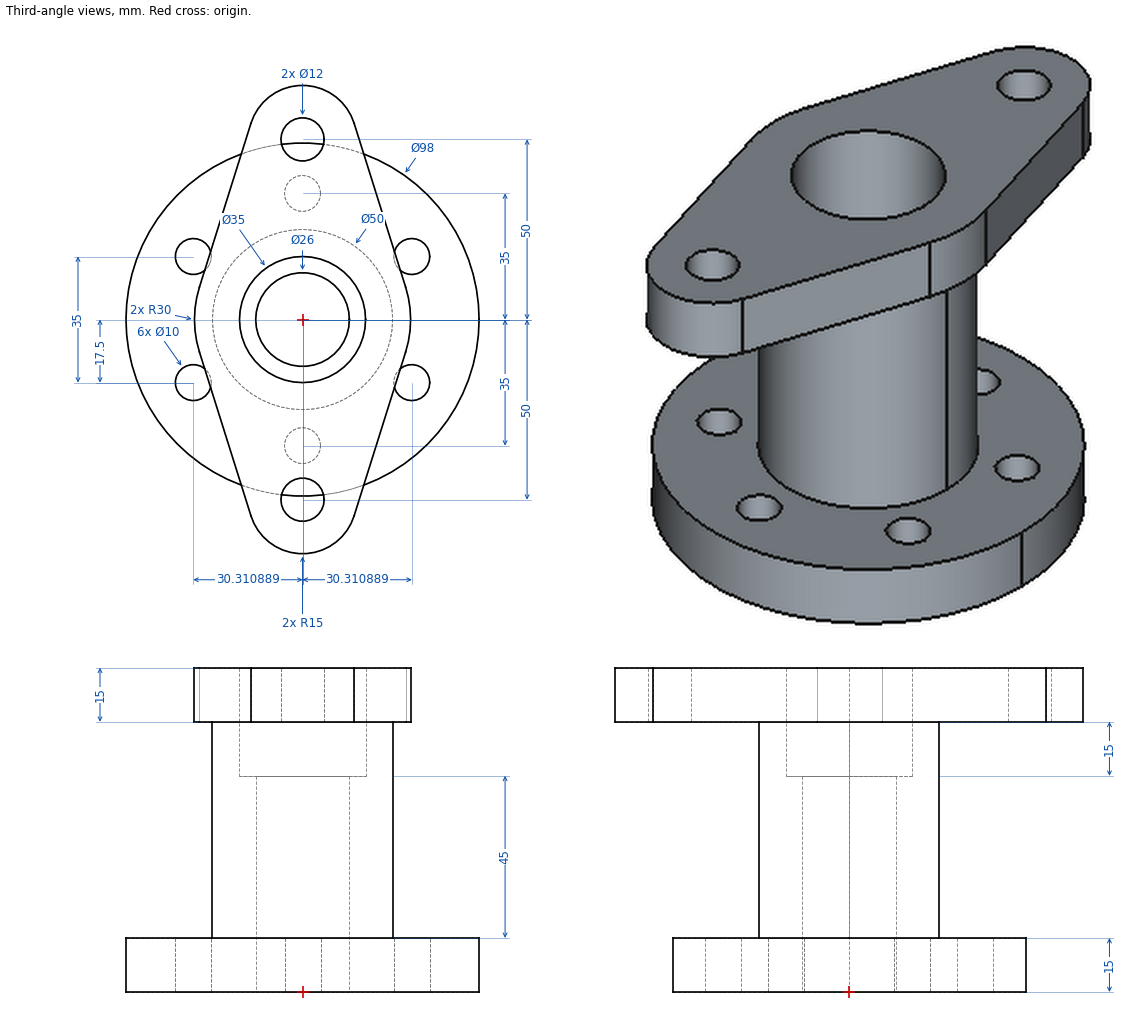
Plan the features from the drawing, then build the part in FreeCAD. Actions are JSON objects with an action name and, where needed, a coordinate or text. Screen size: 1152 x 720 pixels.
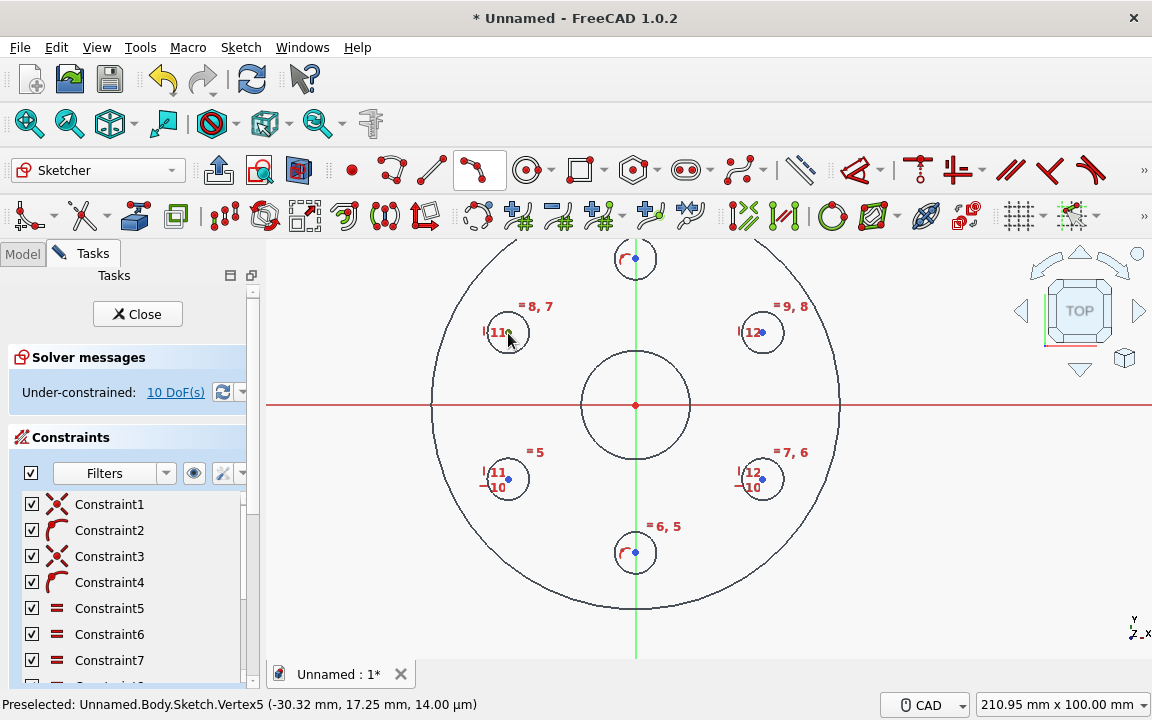
{"action": "left_click", "coordinate": [763, 333]}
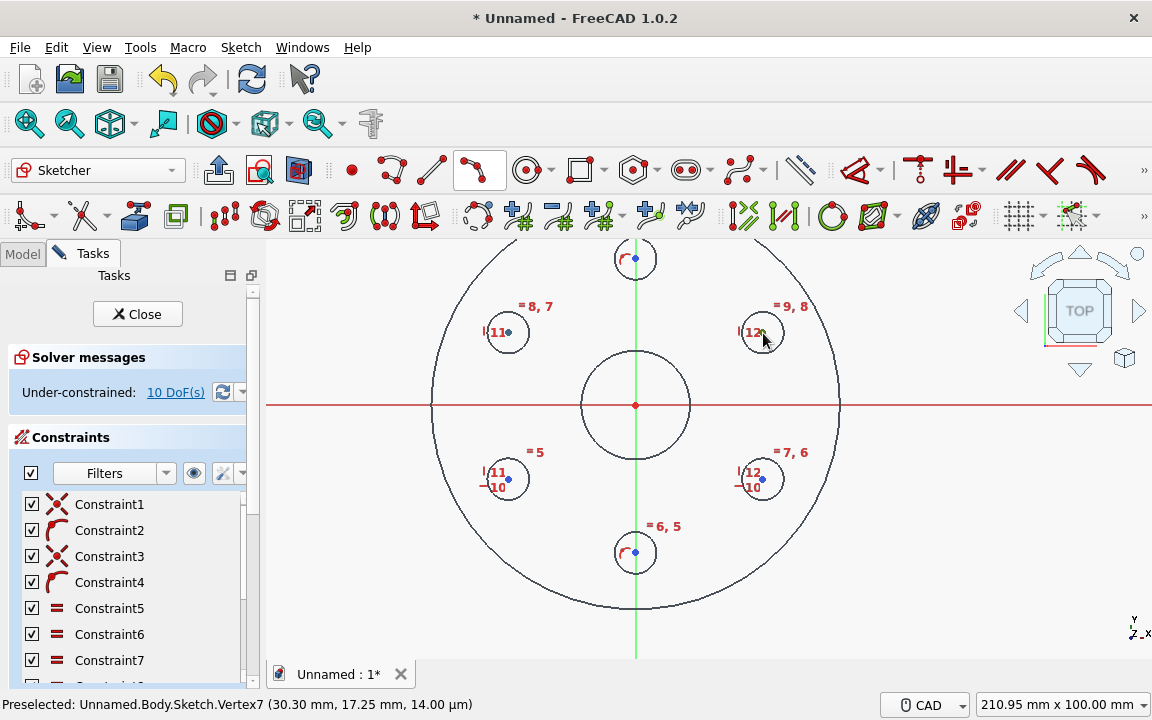
{"action": "key", "text": "h"}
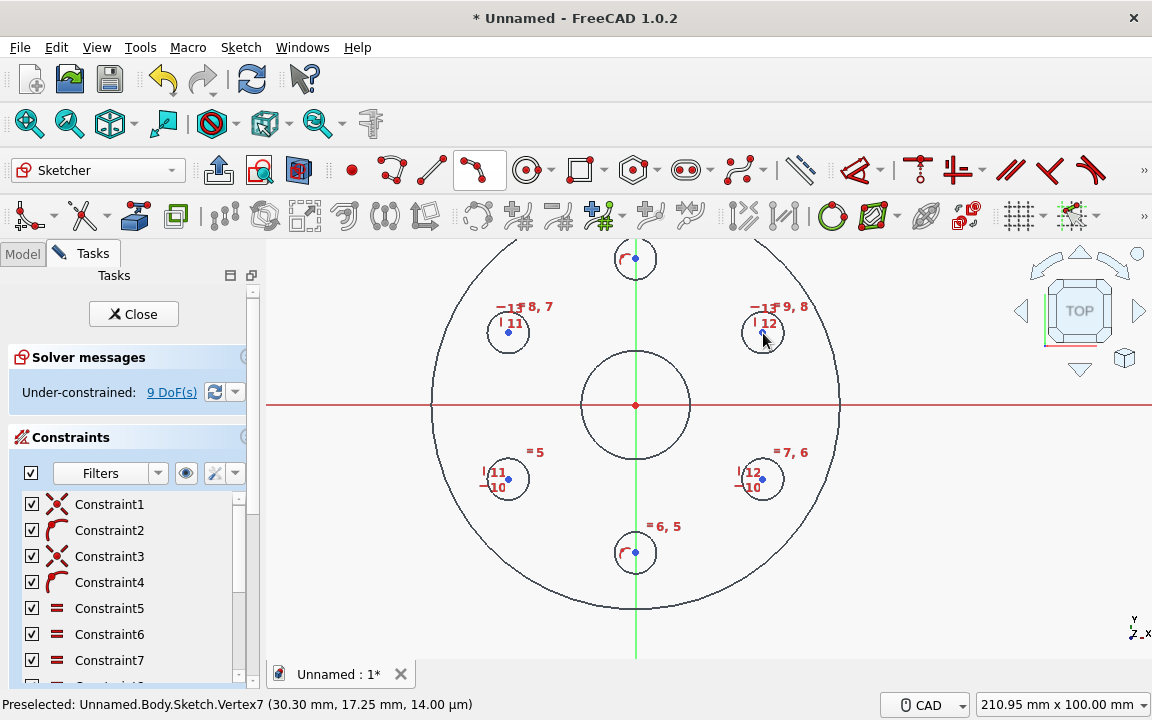
{"action": "left_click", "coordinate": [492, 550]}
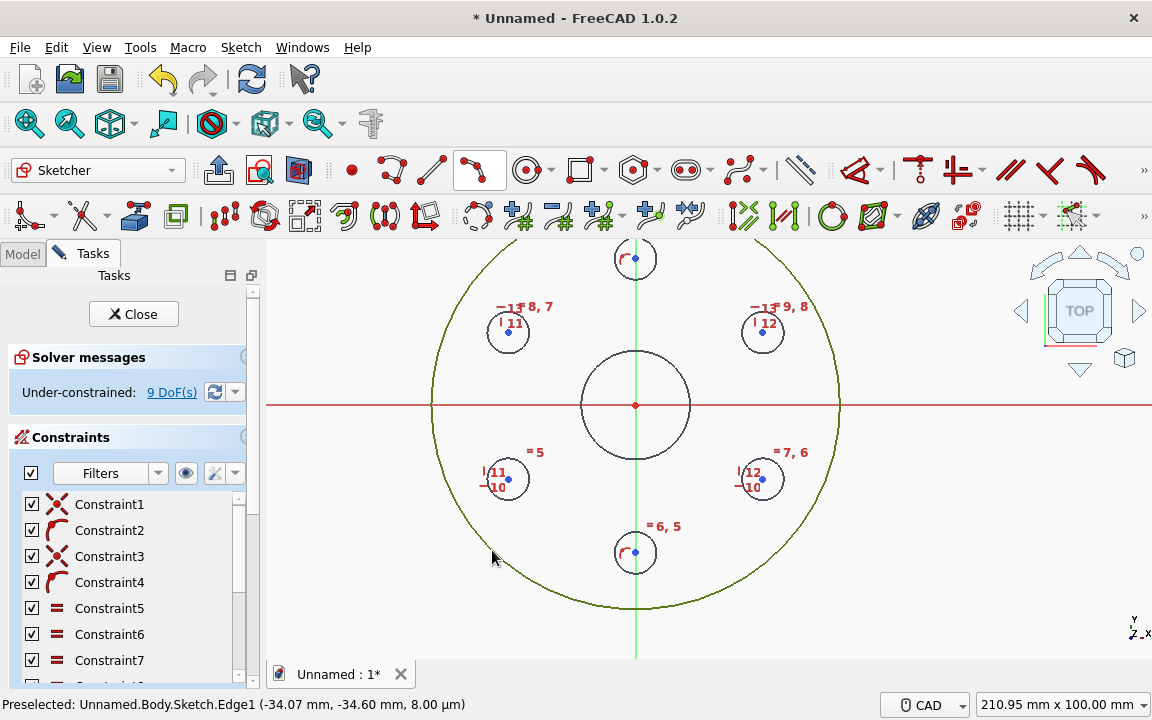
{"action": "key", "text": "k o"}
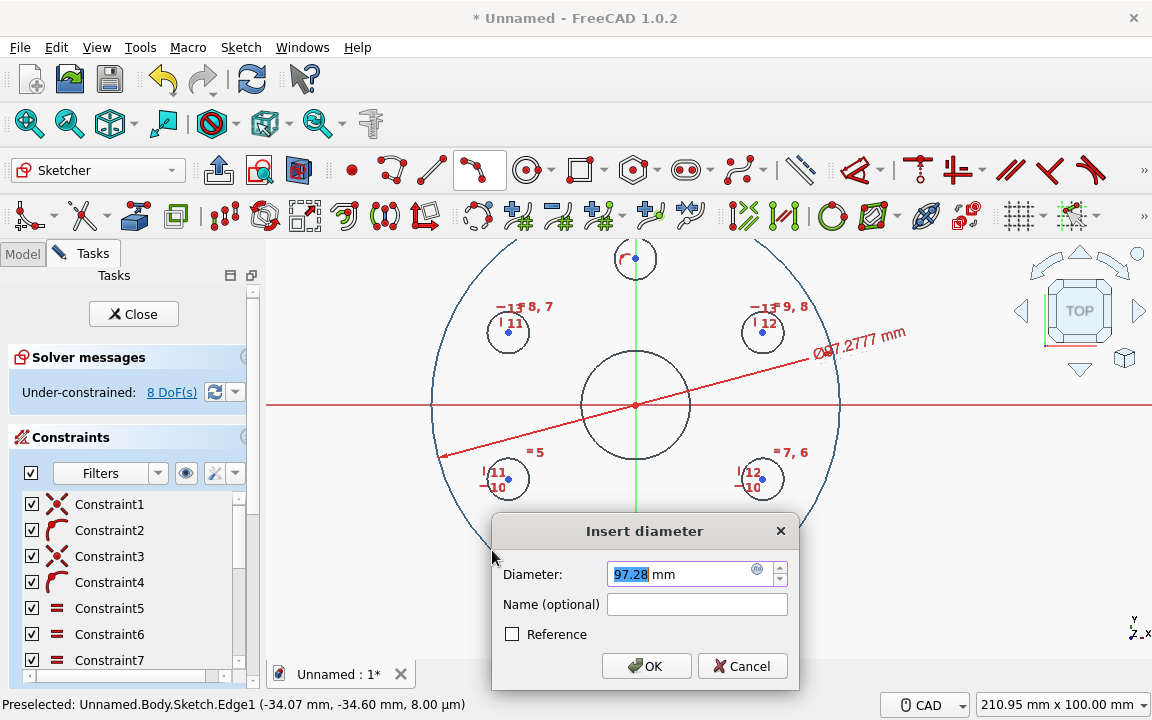
{"action": "type", "text": "98"}
{"action": "key", "text": "Return"}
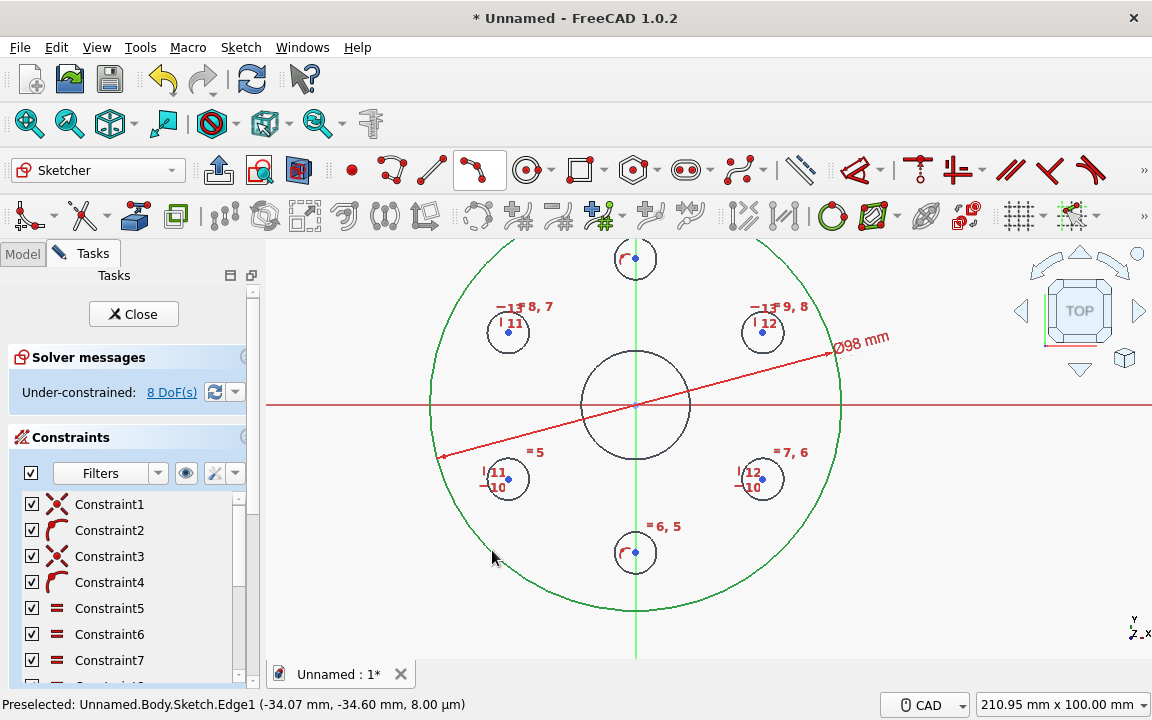
{"action": "left_click", "coordinate": [523, 464]}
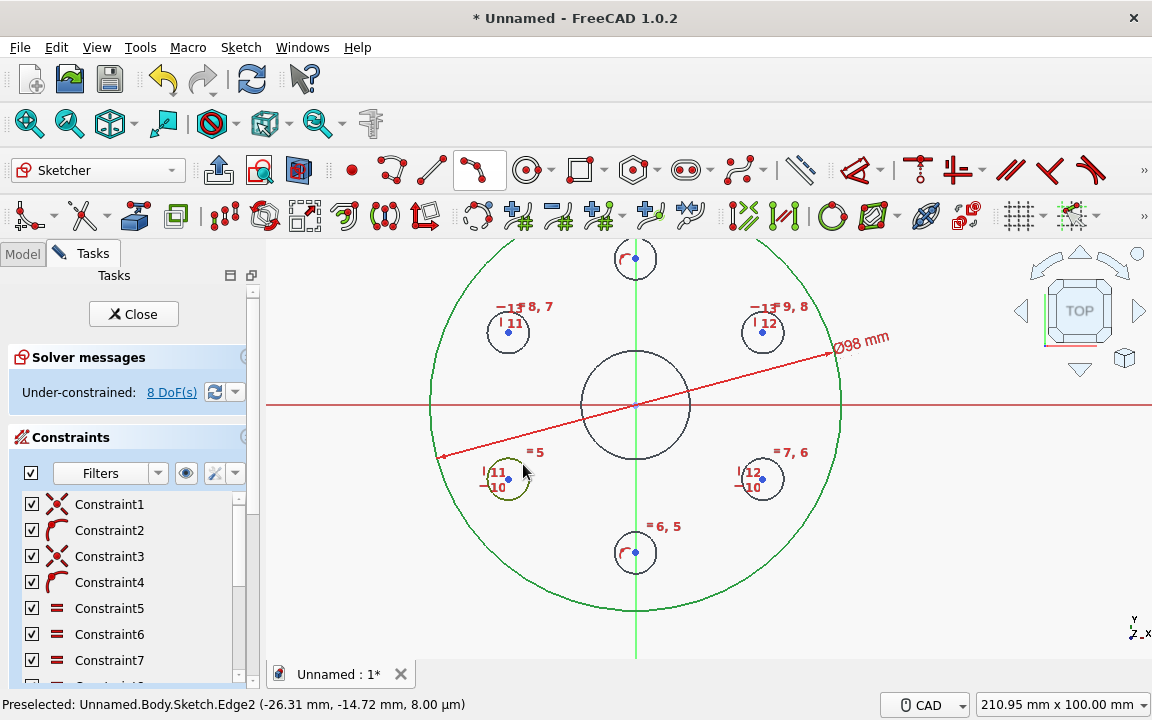
{"action": "key", "text": "k o"}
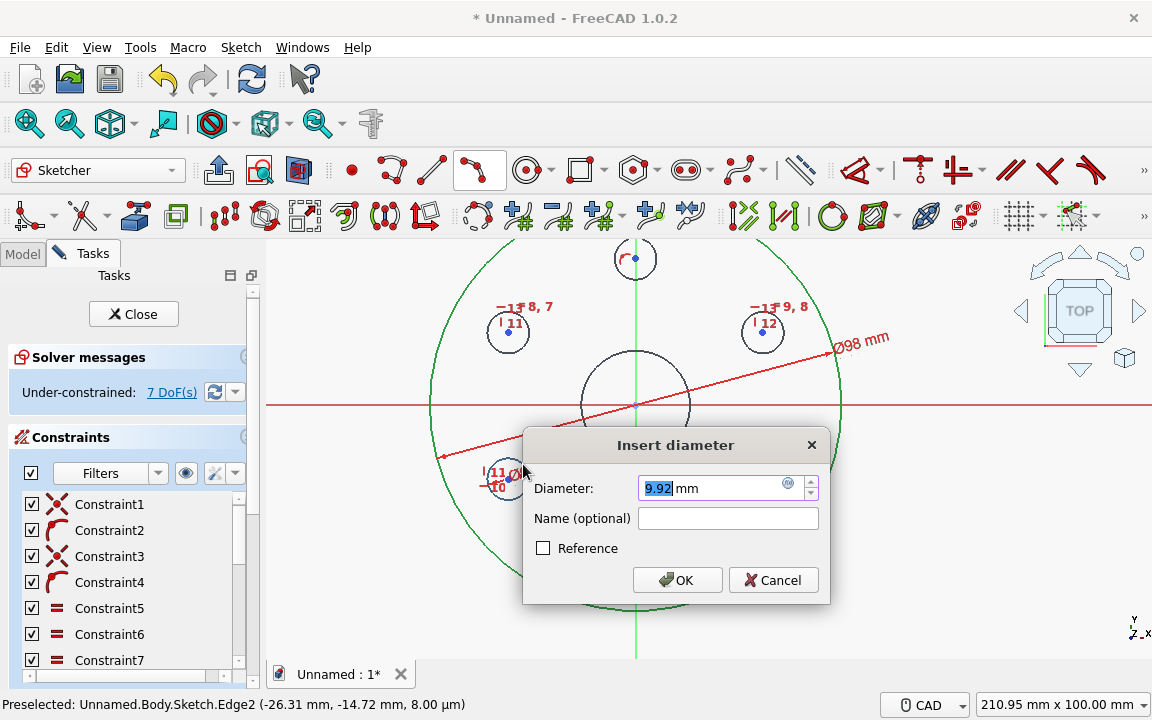
{"action": "type", "text": "10"}
{"action": "key", "text": "Return"}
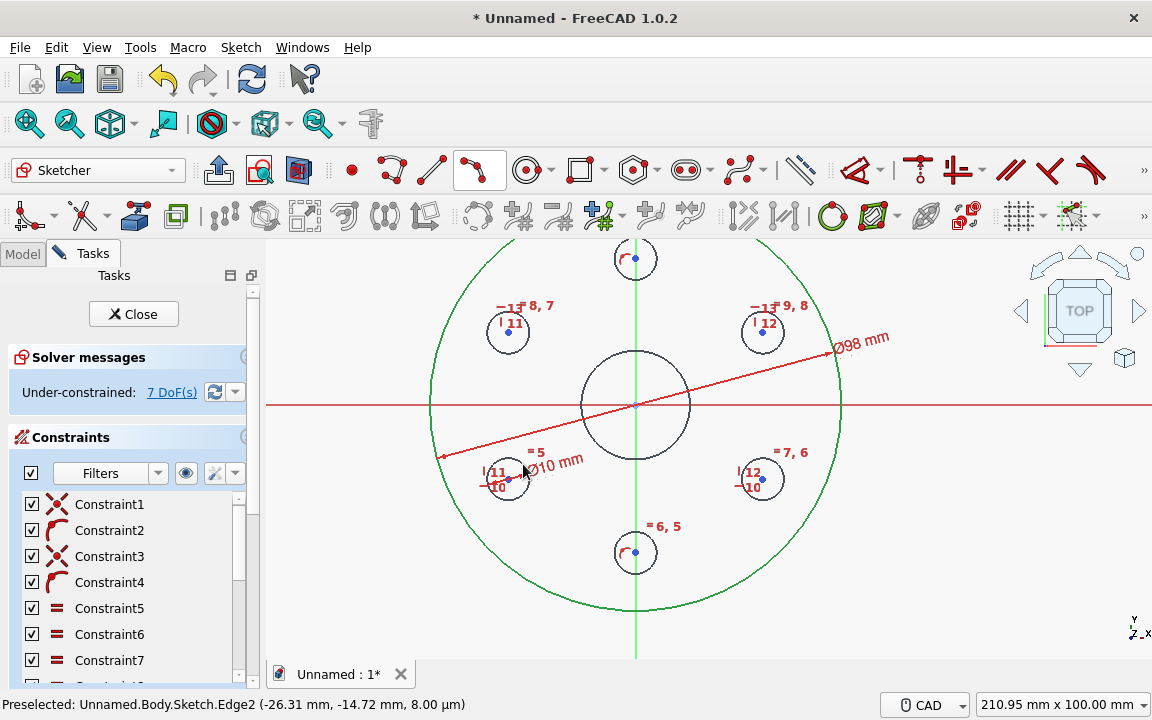
{"action": "left_click", "coordinate": [674, 367]}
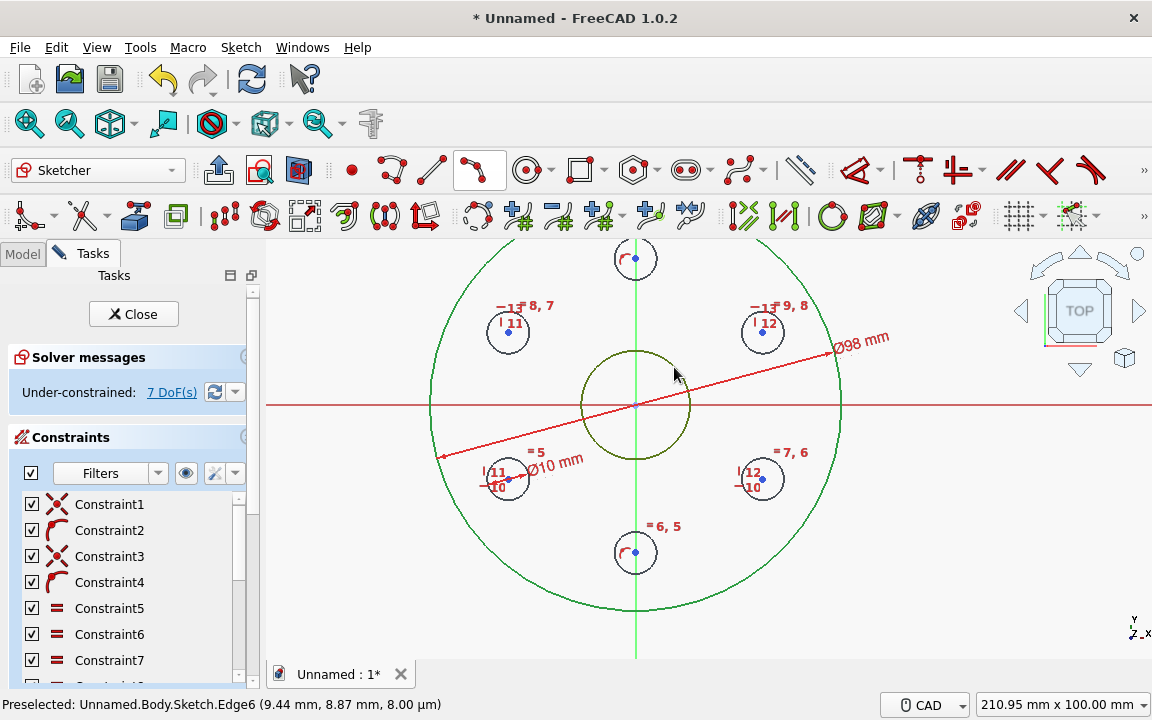
{"action": "key", "text": "k o"}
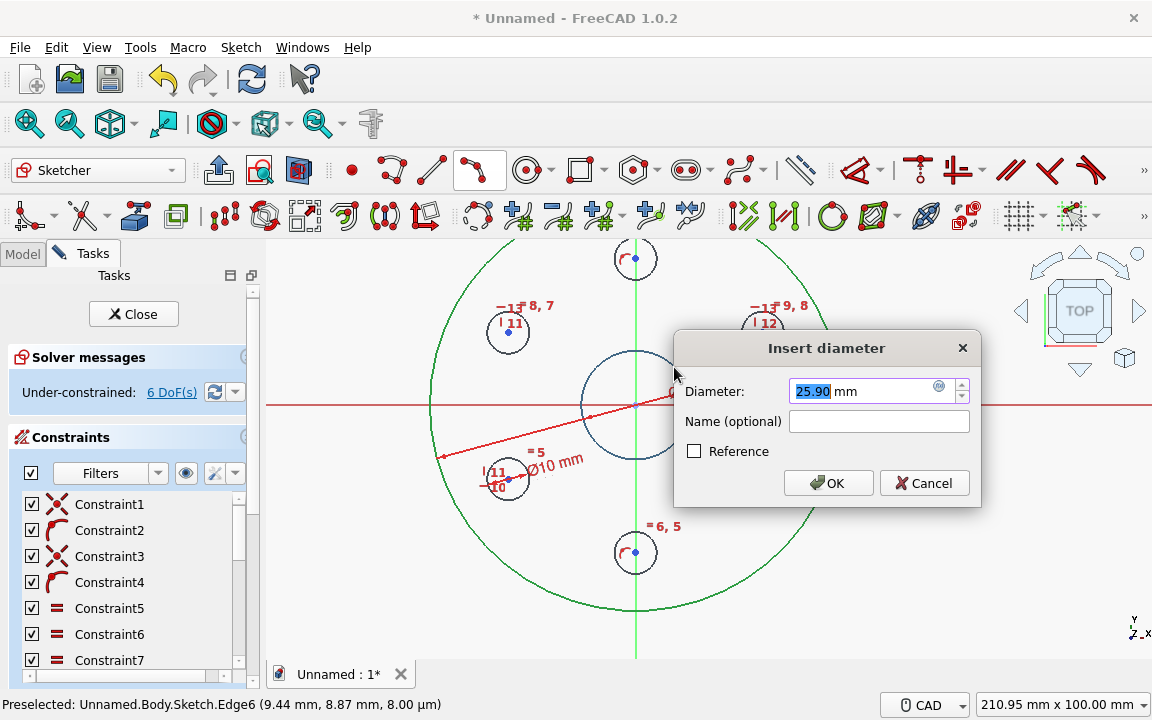
{"action": "type", "text": "26"}
{"action": "key", "text": "Return"}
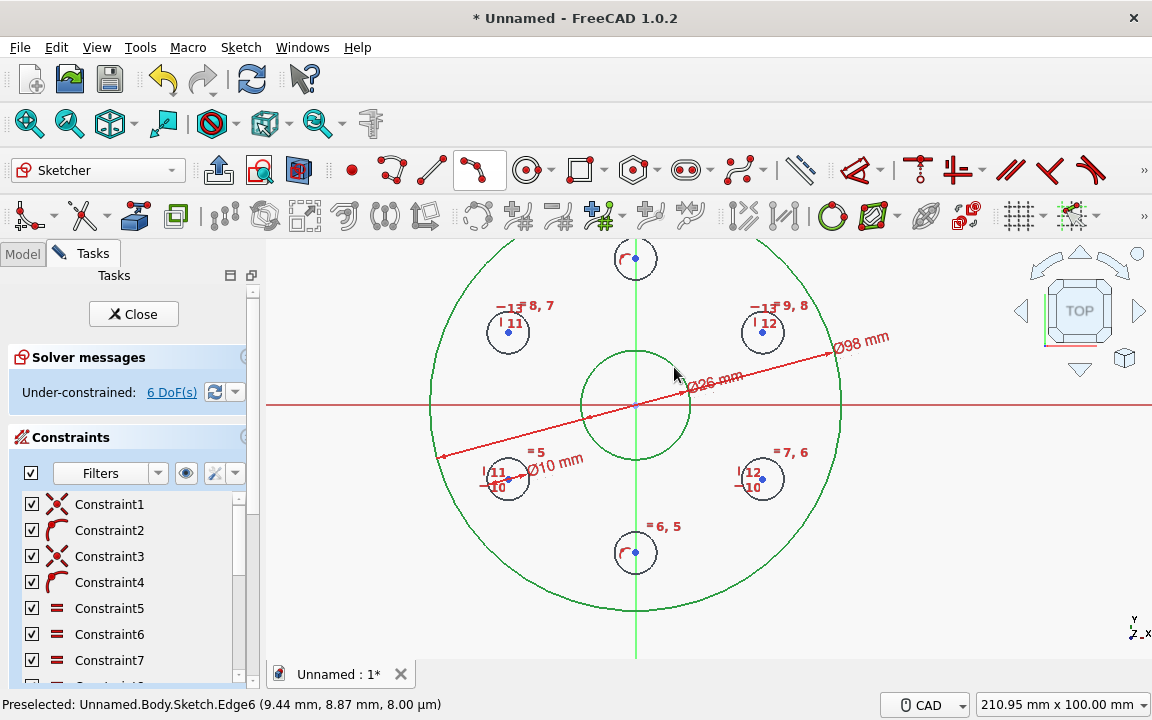
{"action": "left_click", "coordinate": [636, 553]}